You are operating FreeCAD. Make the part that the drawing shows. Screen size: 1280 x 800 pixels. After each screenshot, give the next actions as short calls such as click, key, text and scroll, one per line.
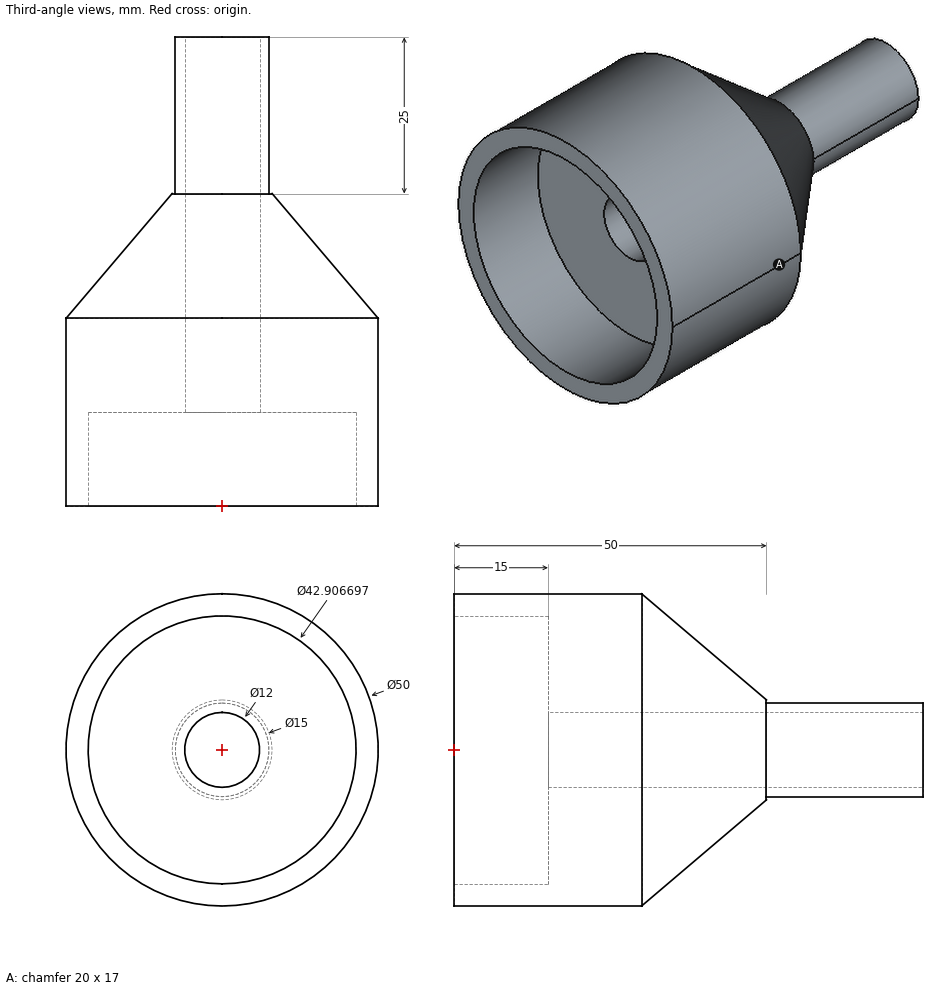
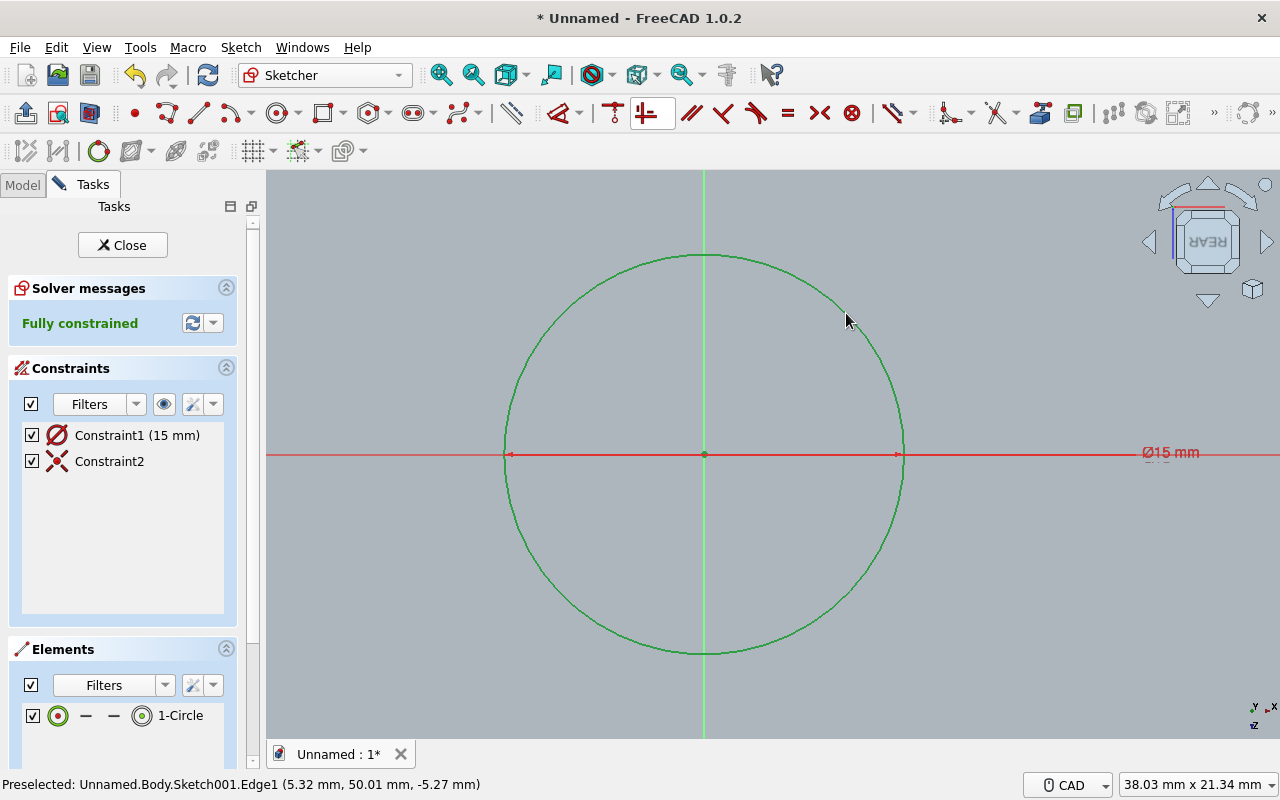
click(123, 245)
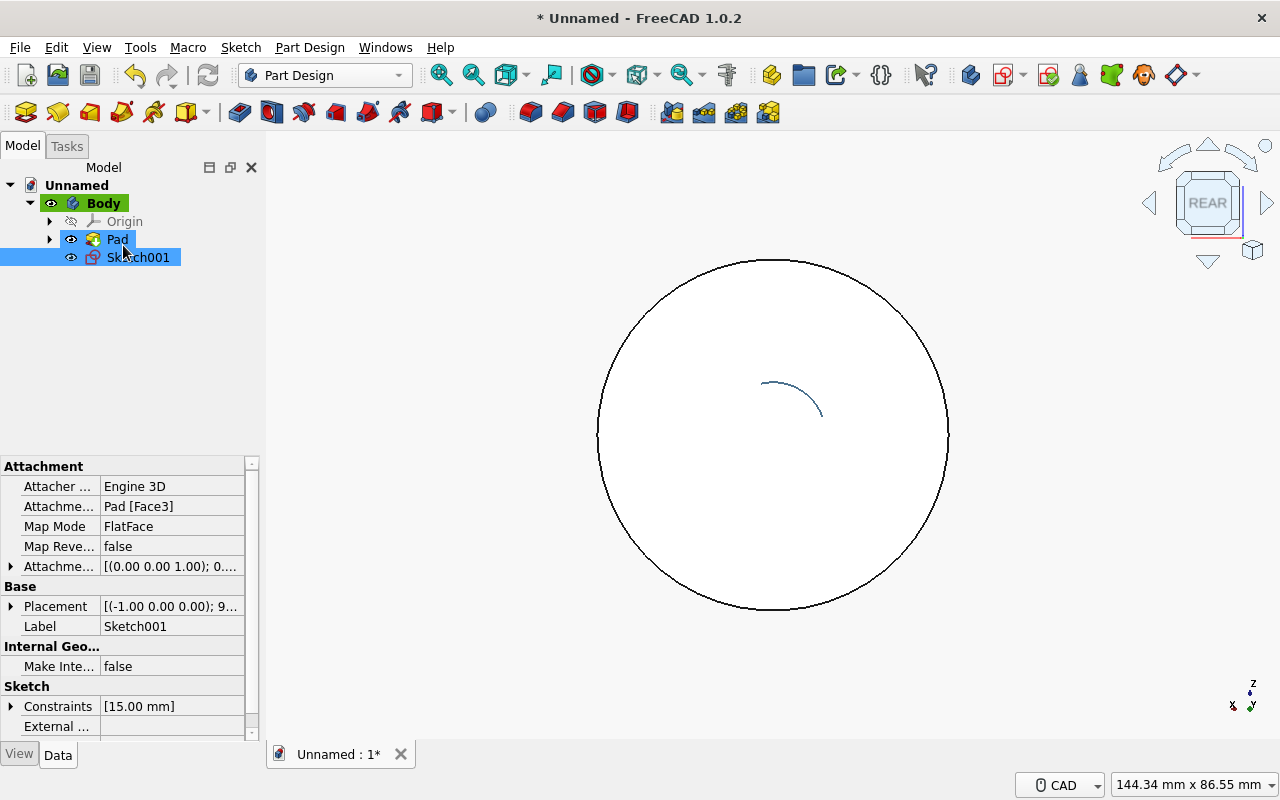
click(26, 112)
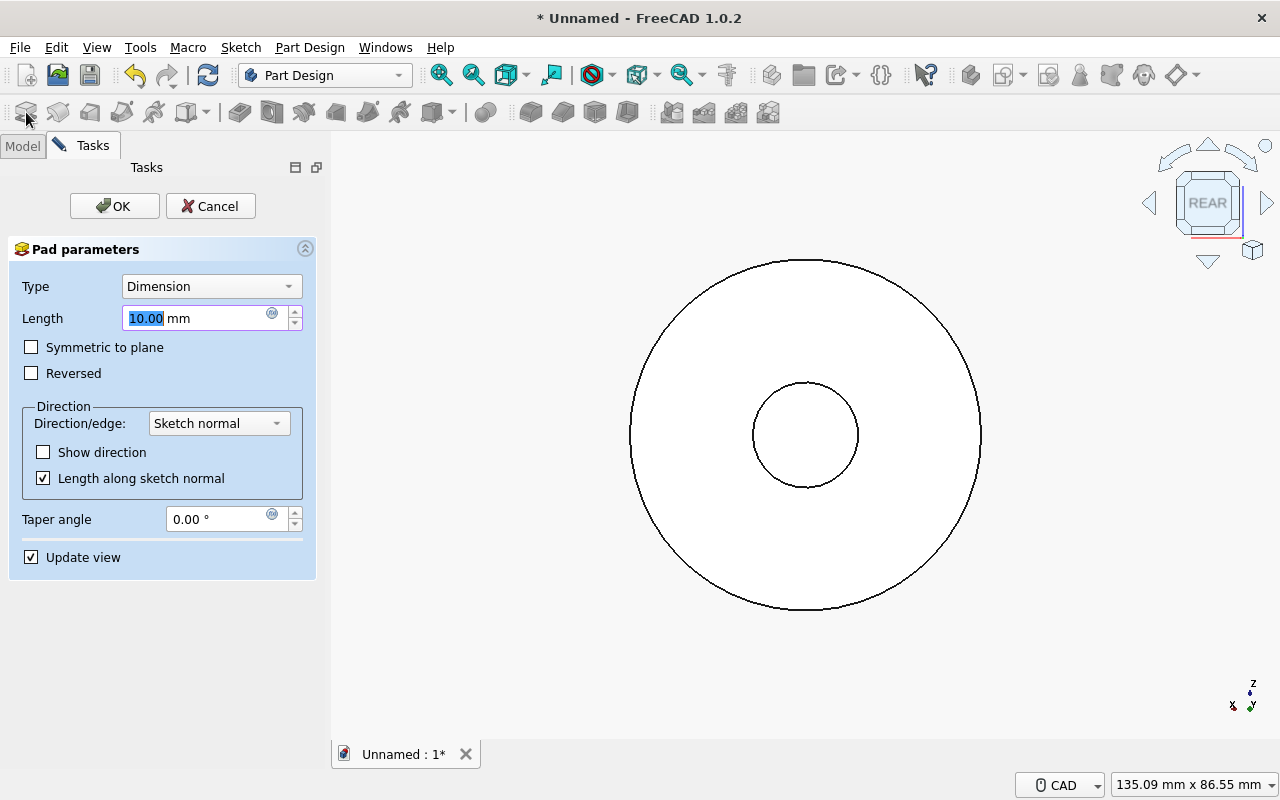
text(25)
key(Tab)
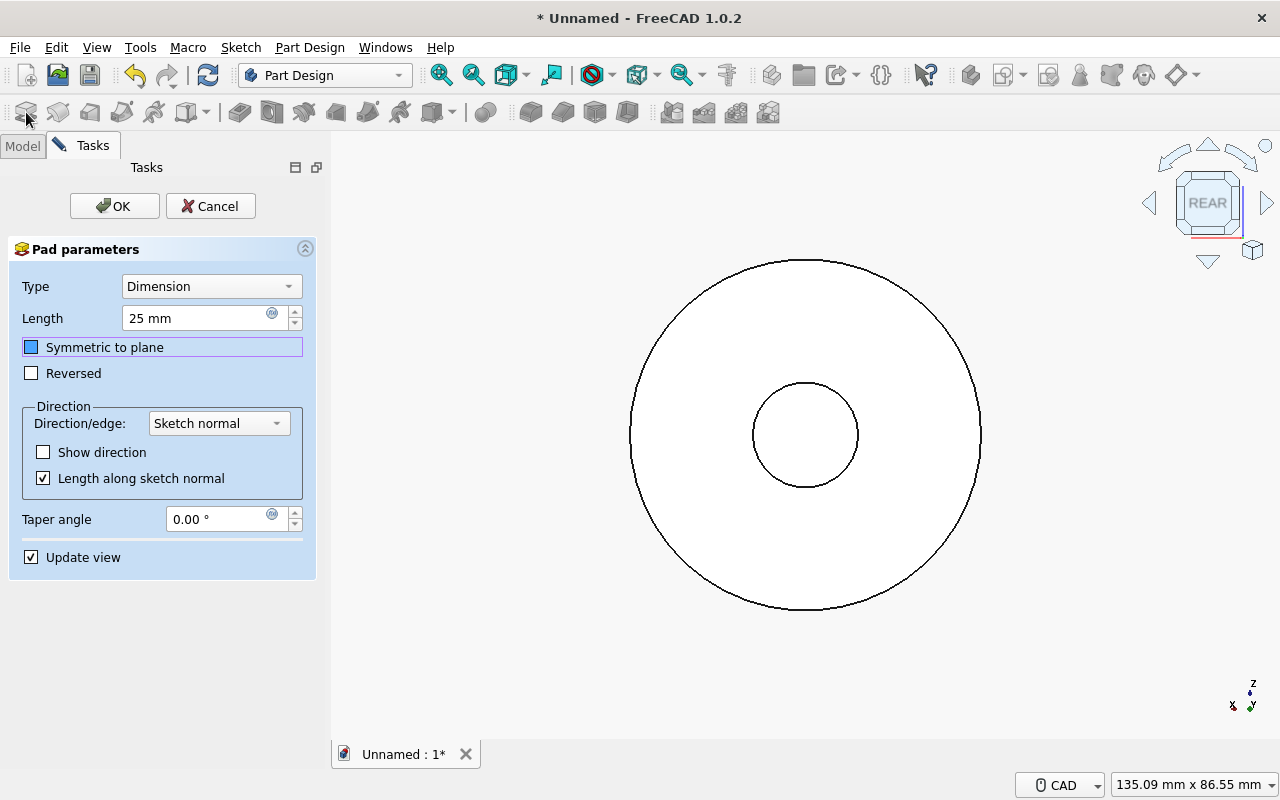
click(115, 206)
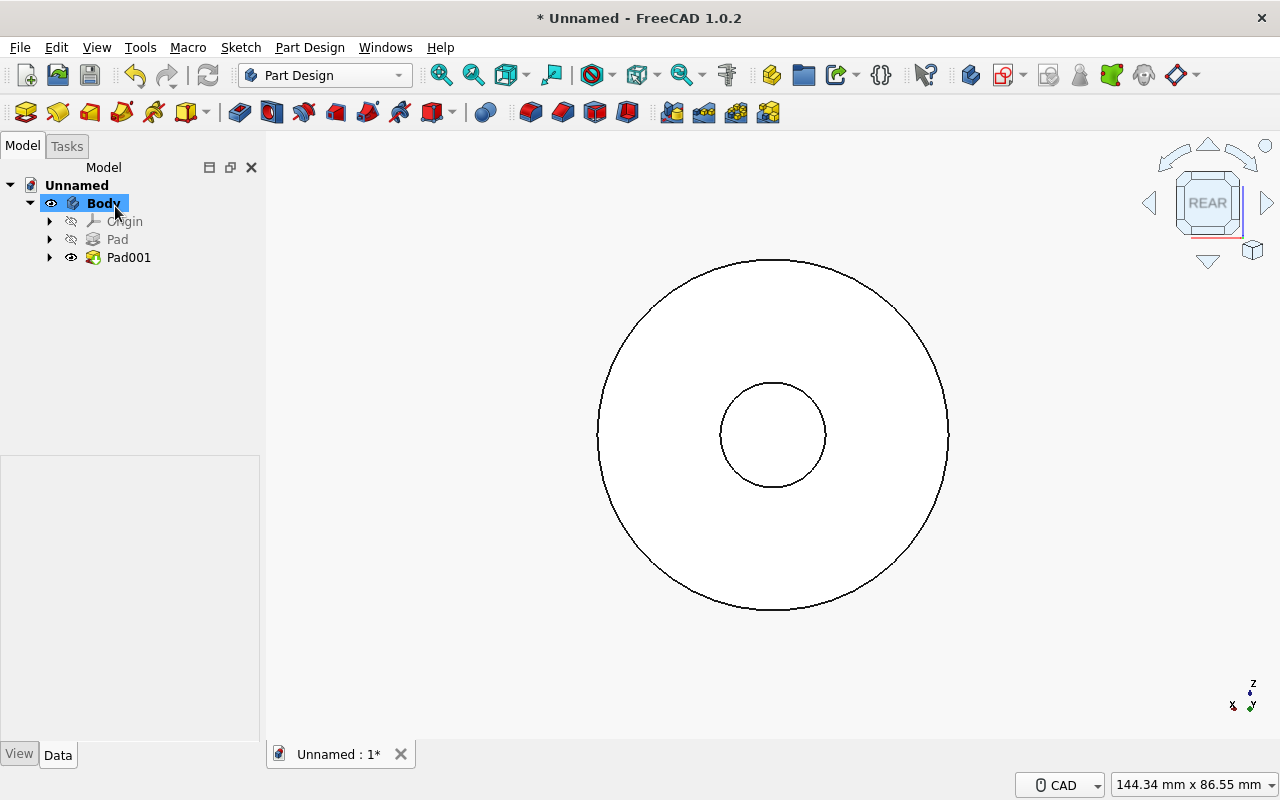
click(949, 434)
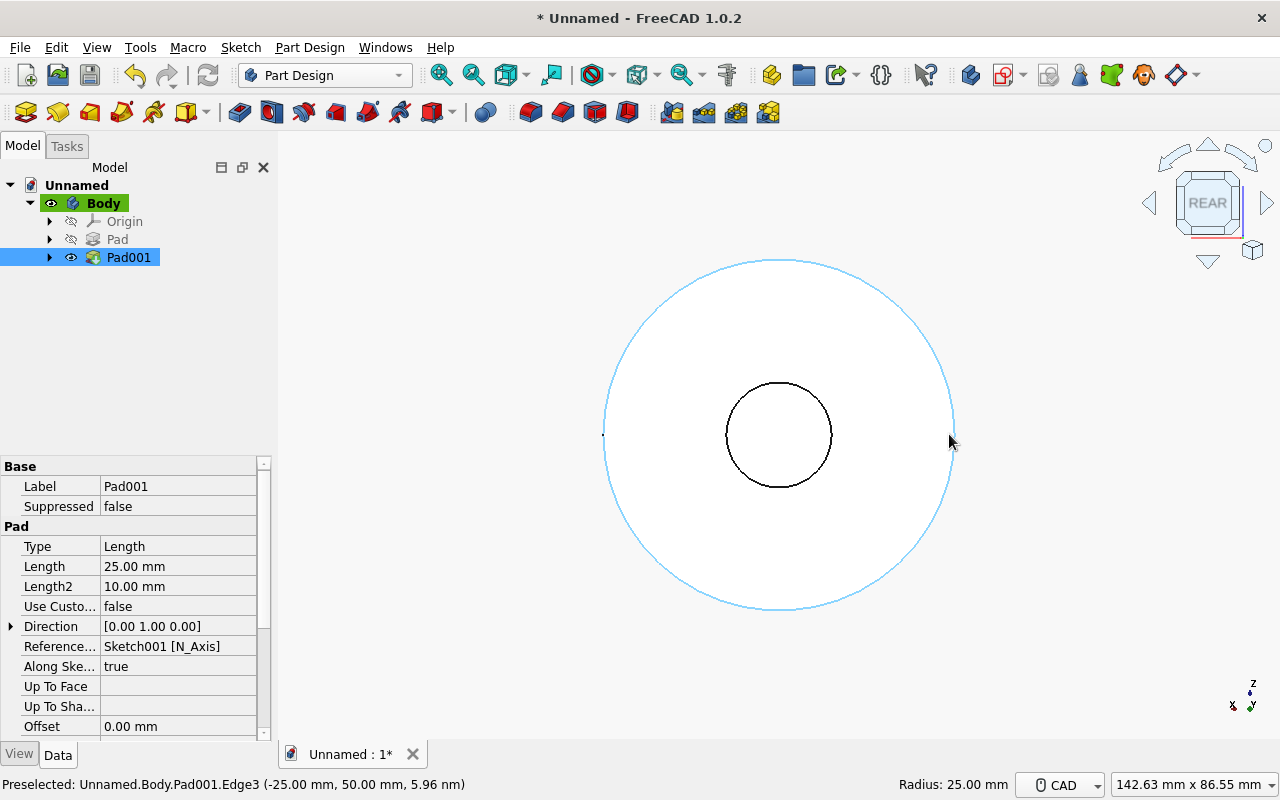
click(564, 112)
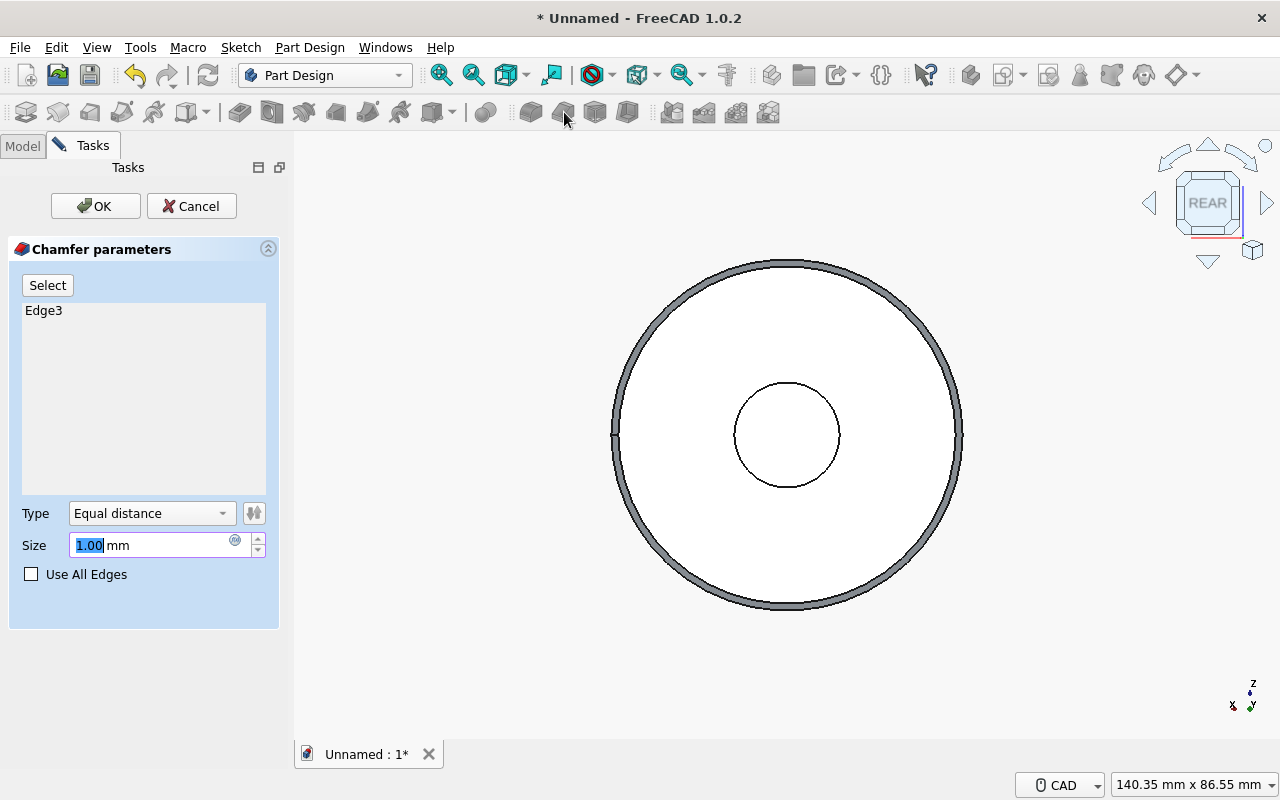
text(20)
key(Tab)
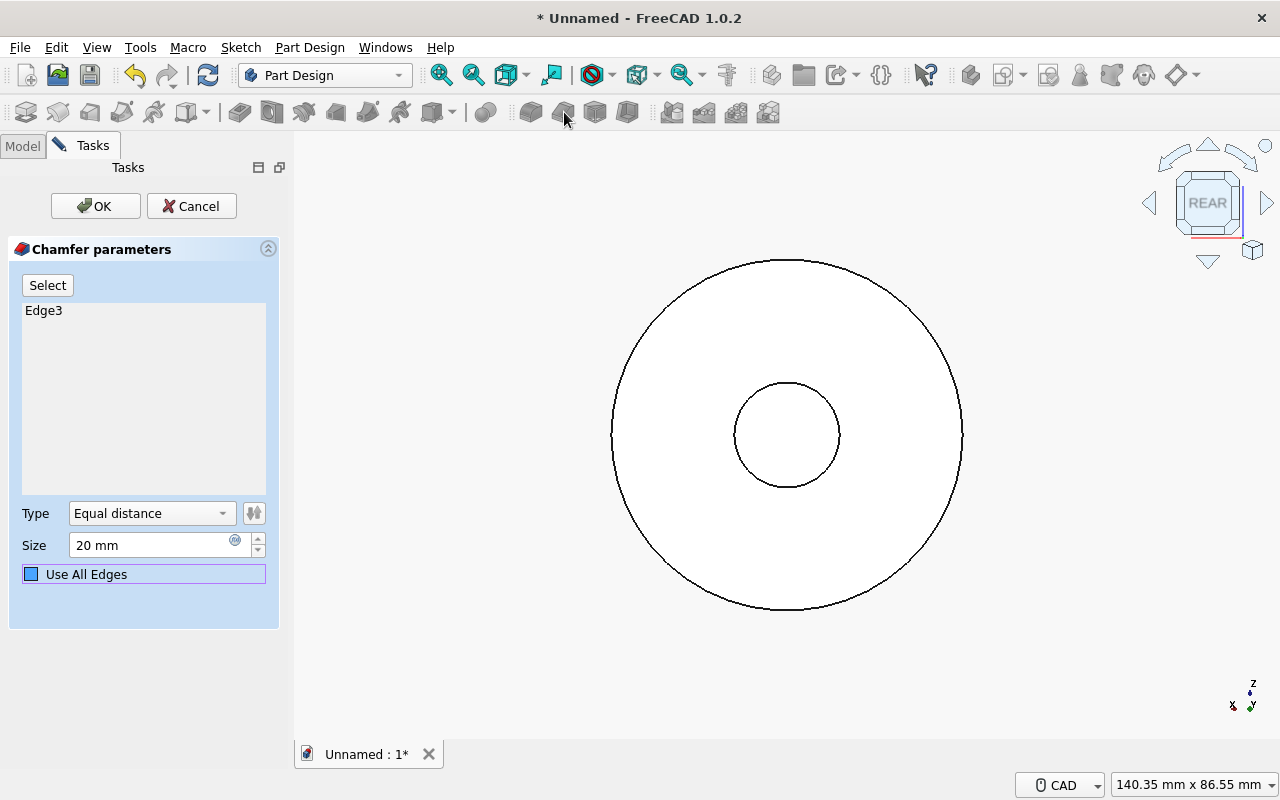
click(153, 514)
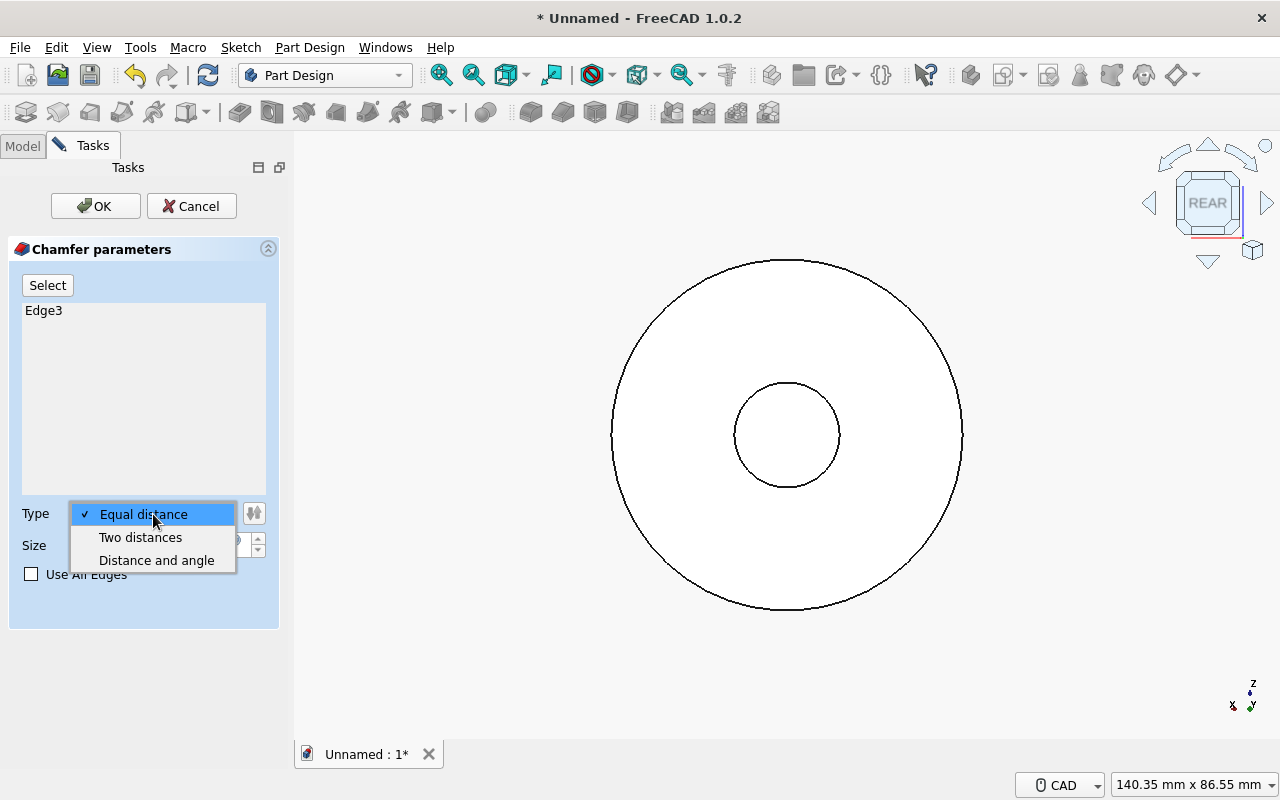
click(152, 538)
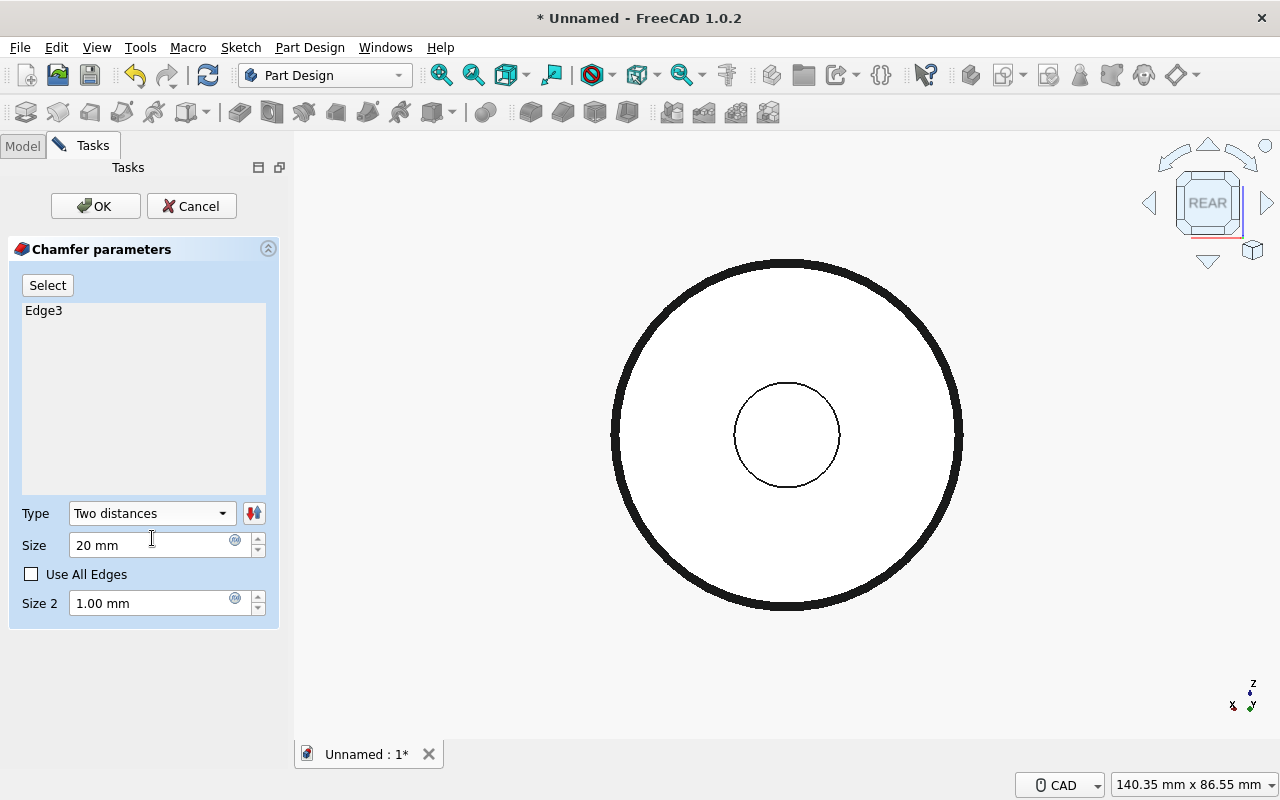
triple_click(160, 603)